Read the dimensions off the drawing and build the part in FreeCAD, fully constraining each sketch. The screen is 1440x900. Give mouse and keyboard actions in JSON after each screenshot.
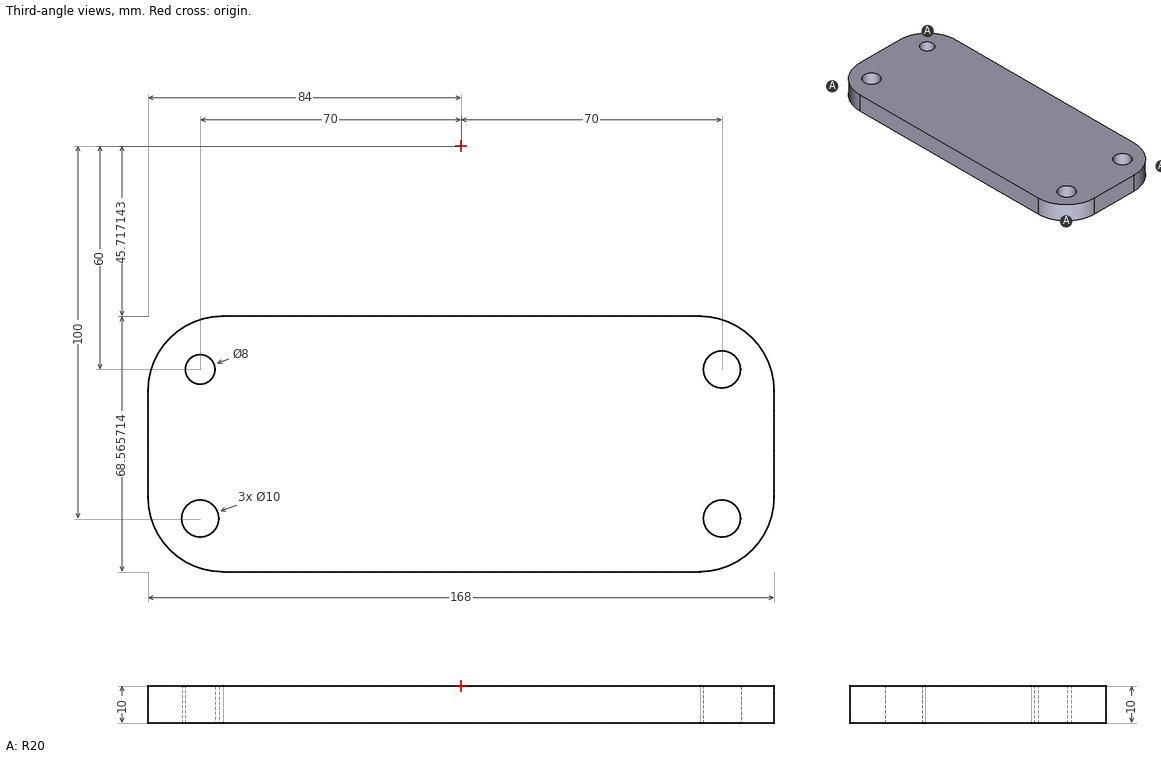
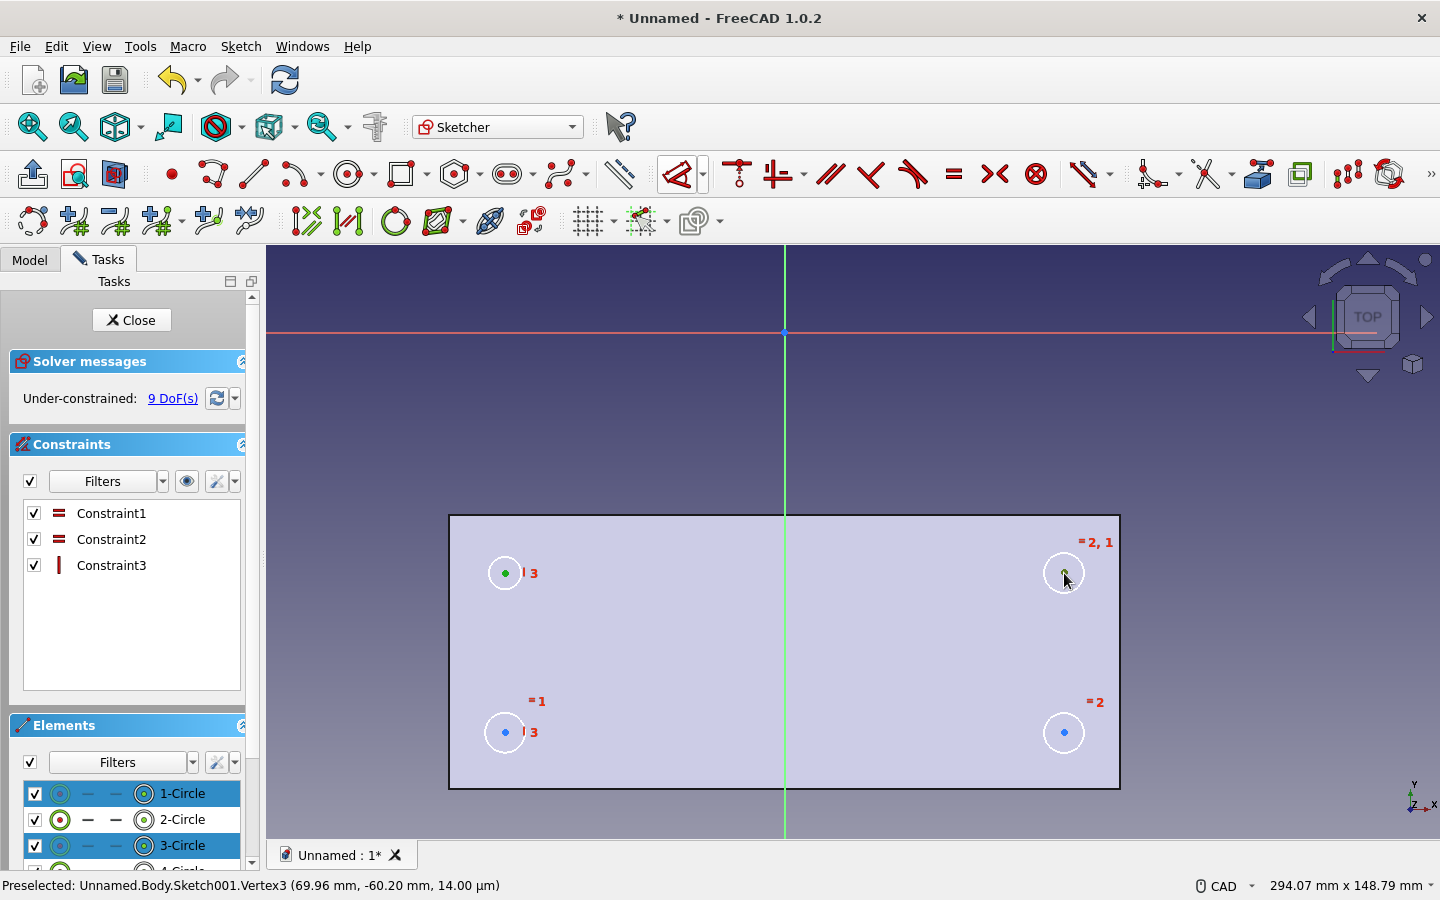
{"action": "key", "text": "h"}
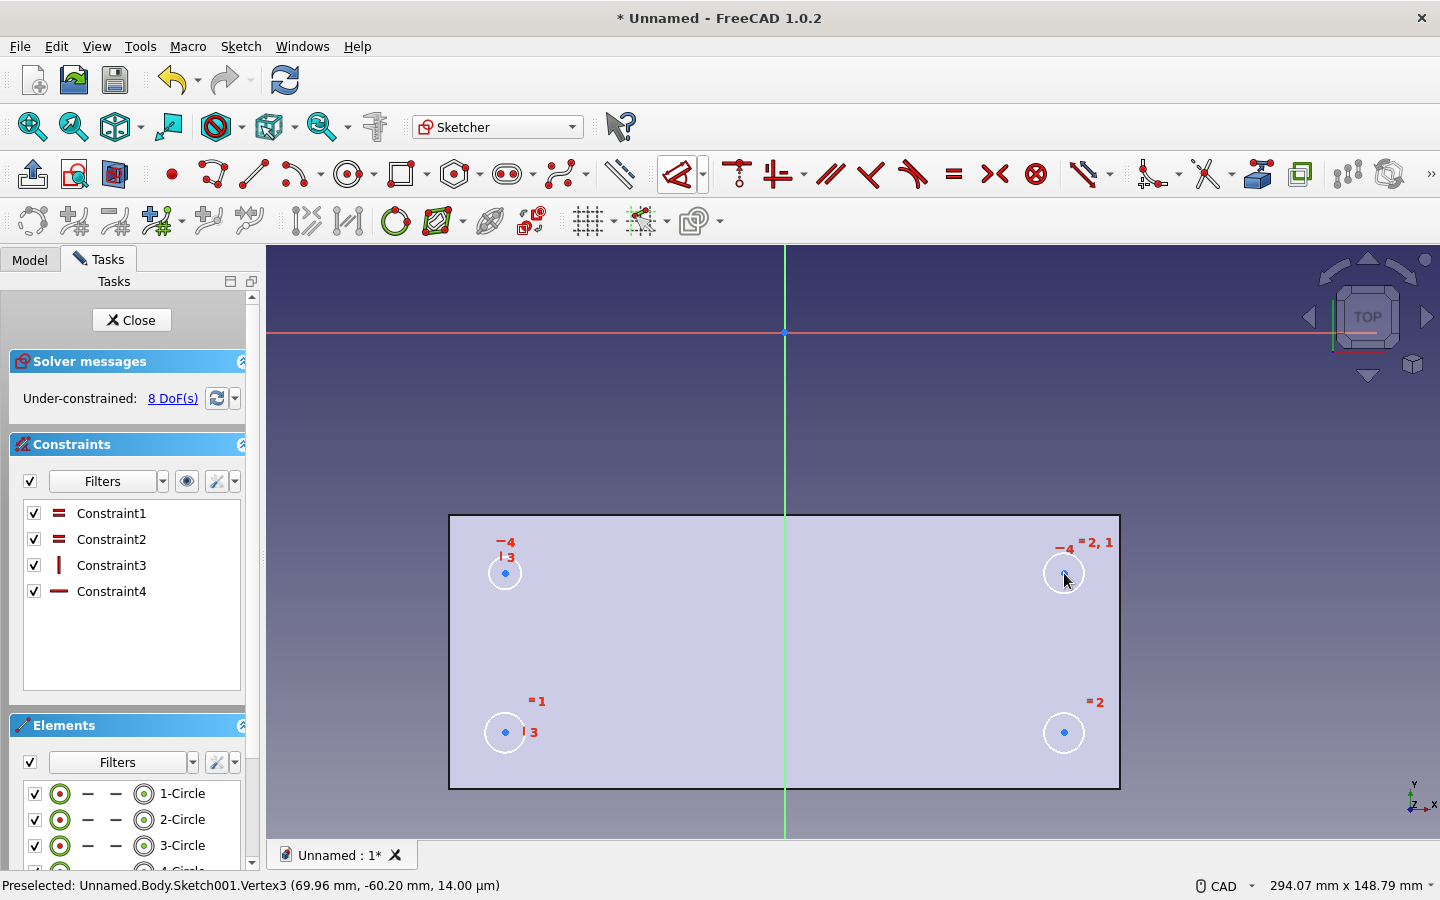
{"action": "left_click", "coordinate": [1064, 573]}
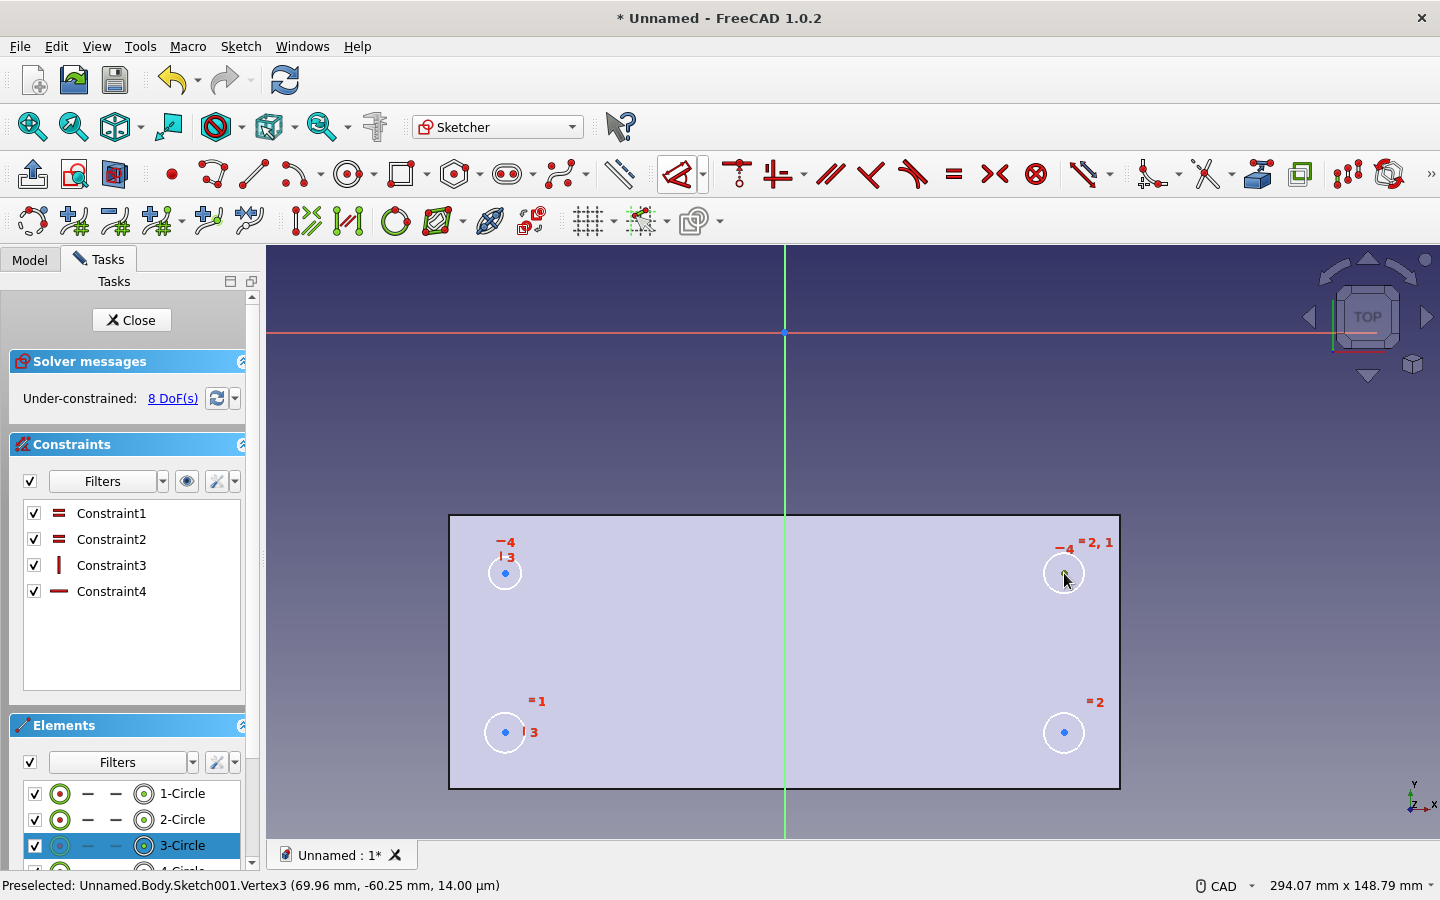
{"action": "left_click", "coordinate": [1064, 733]}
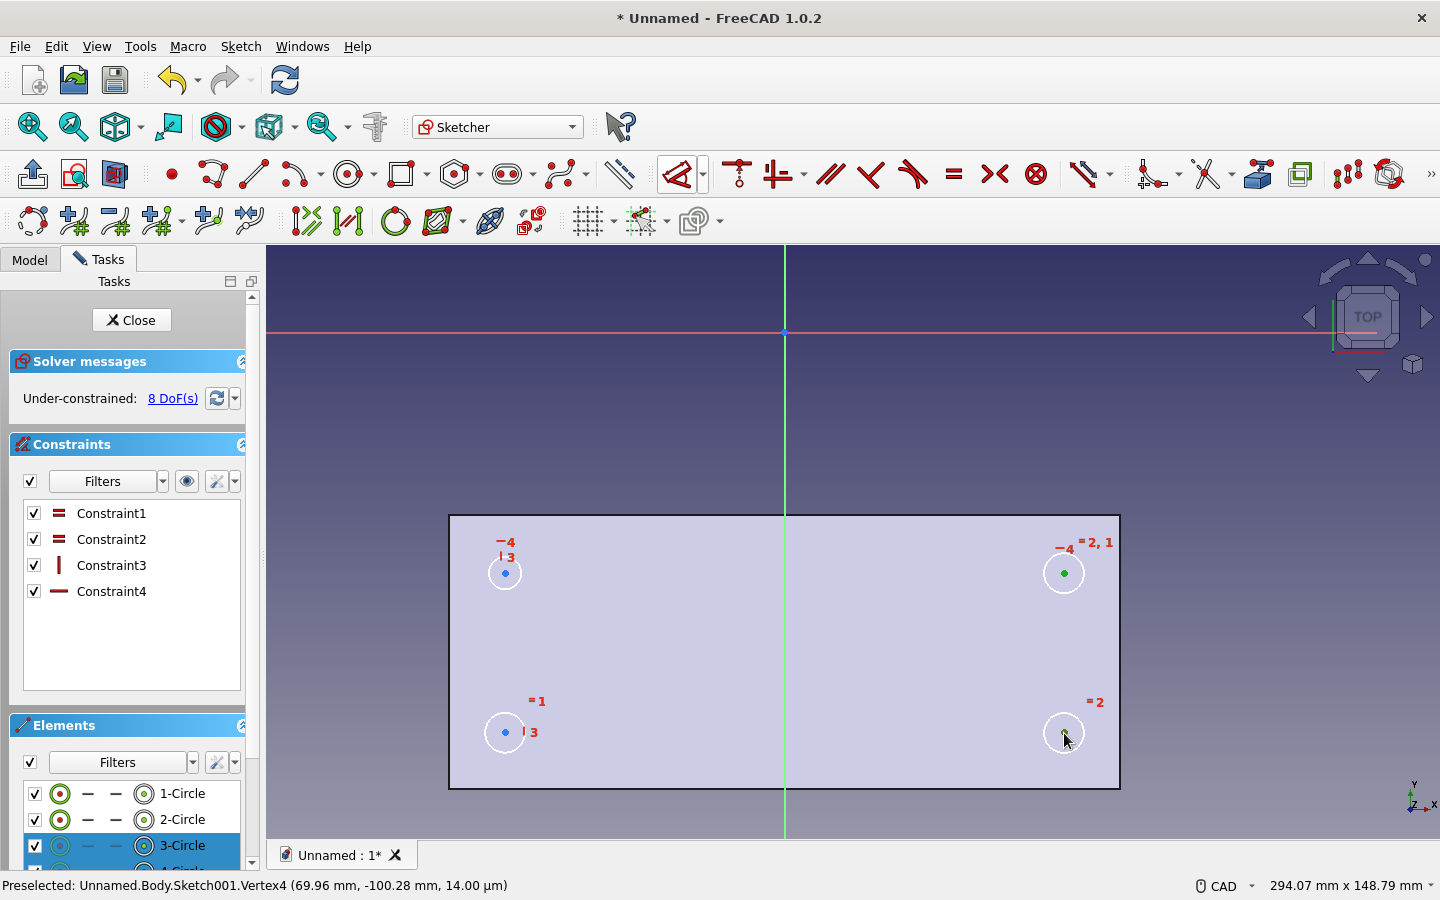
{"action": "key", "text": "v"}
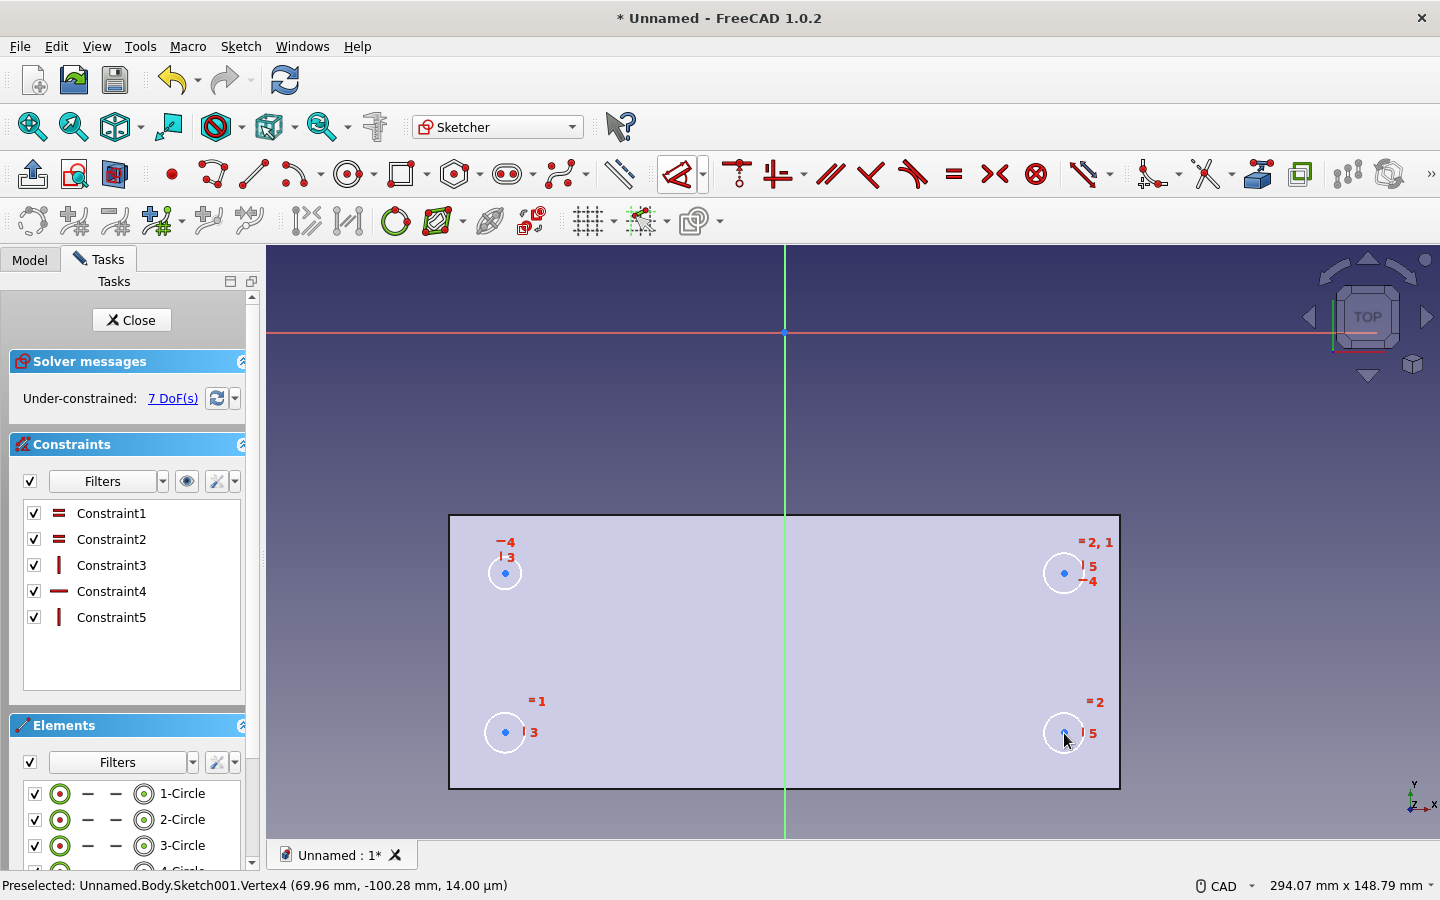
{"action": "left_click", "coordinate": [505, 733]}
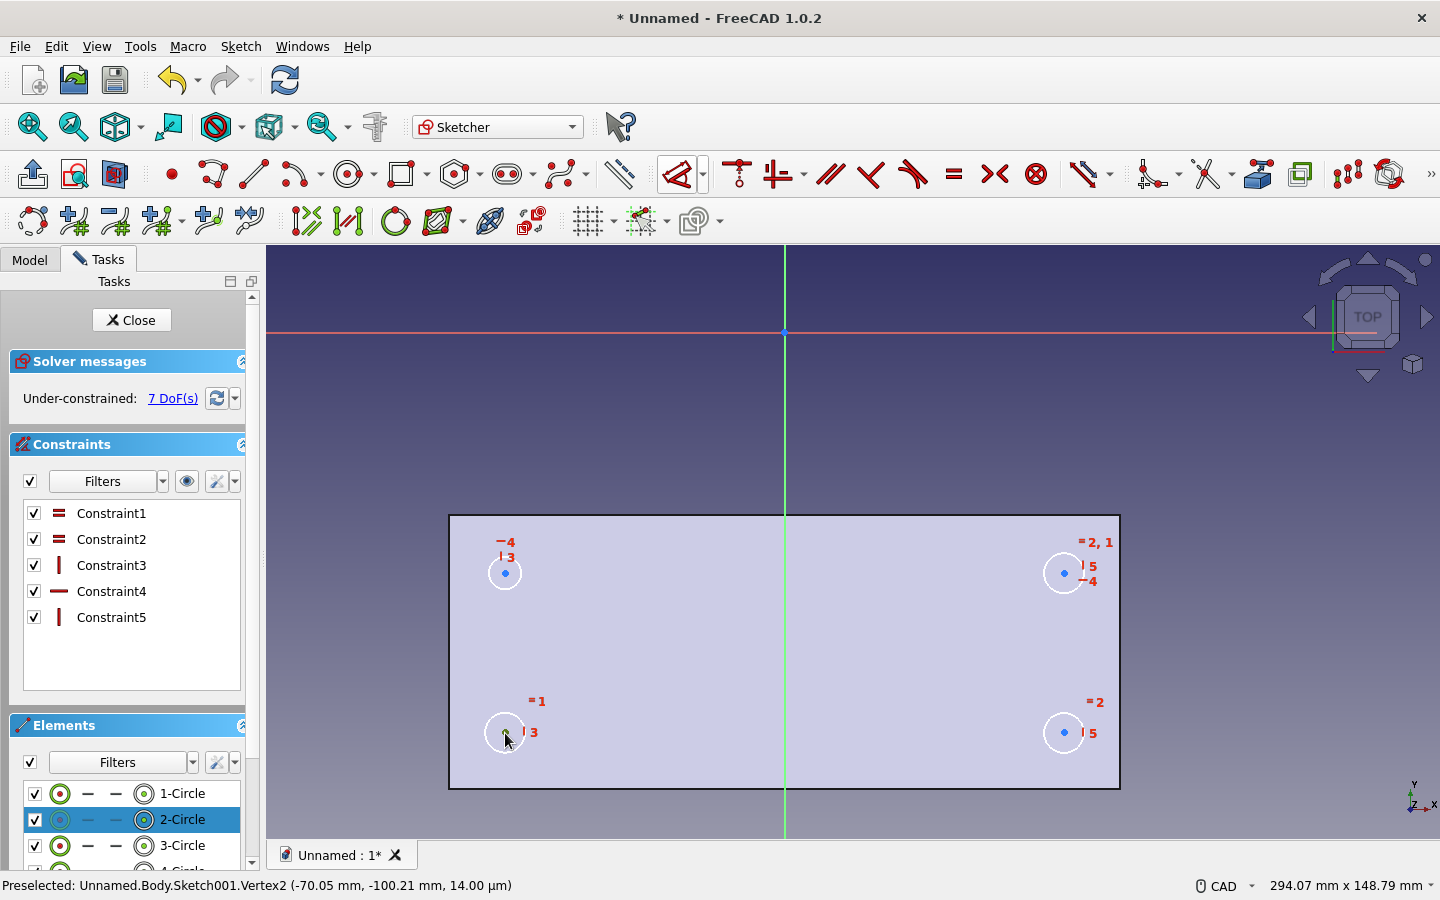
{"action": "left_click", "coordinate": [1064, 733]}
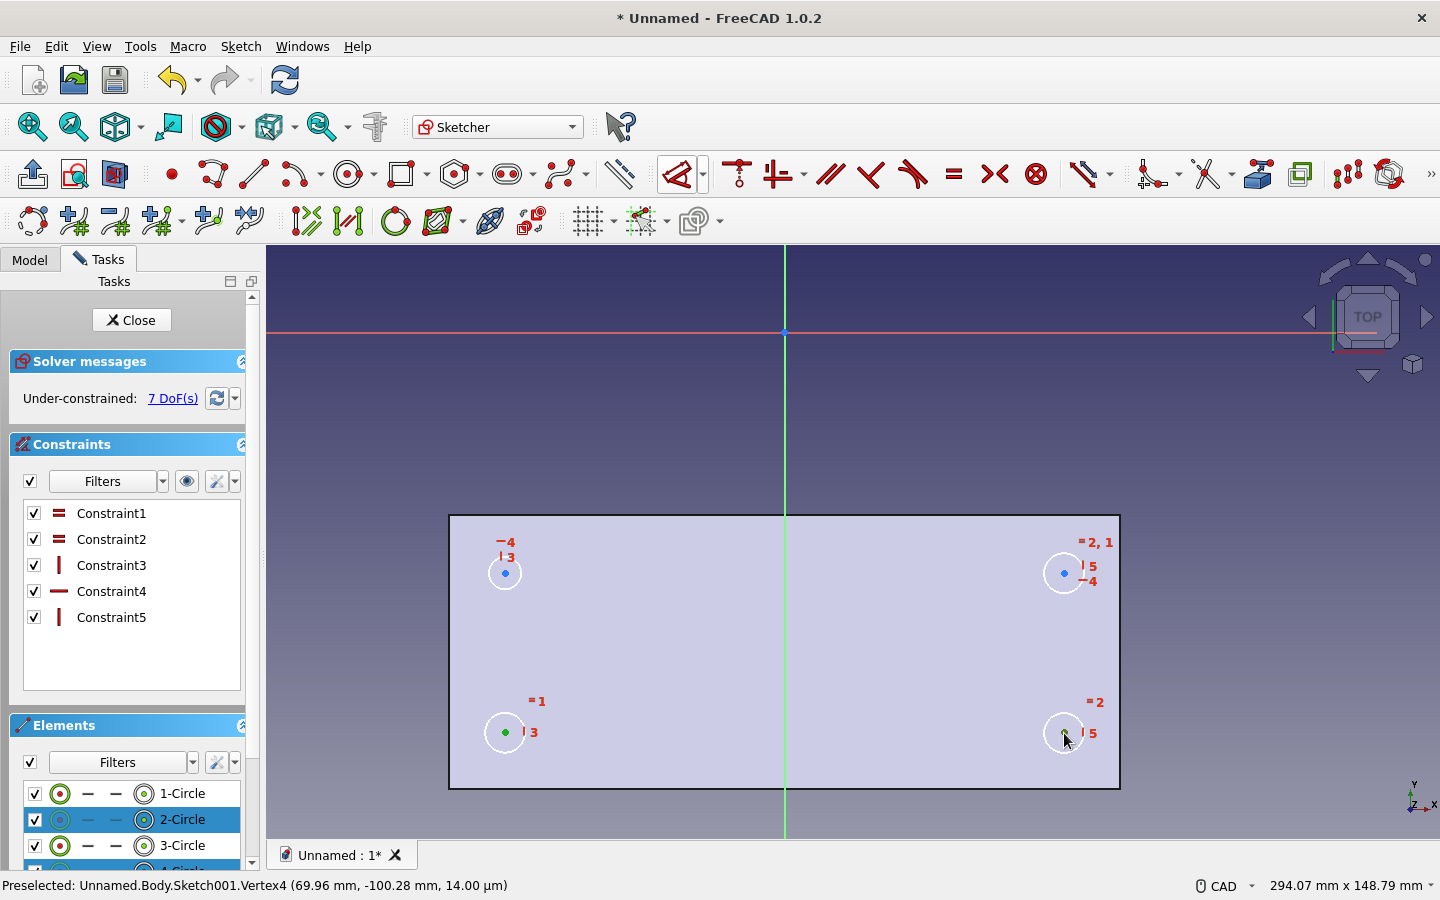
{"action": "left_click", "coordinate": [804, 174]}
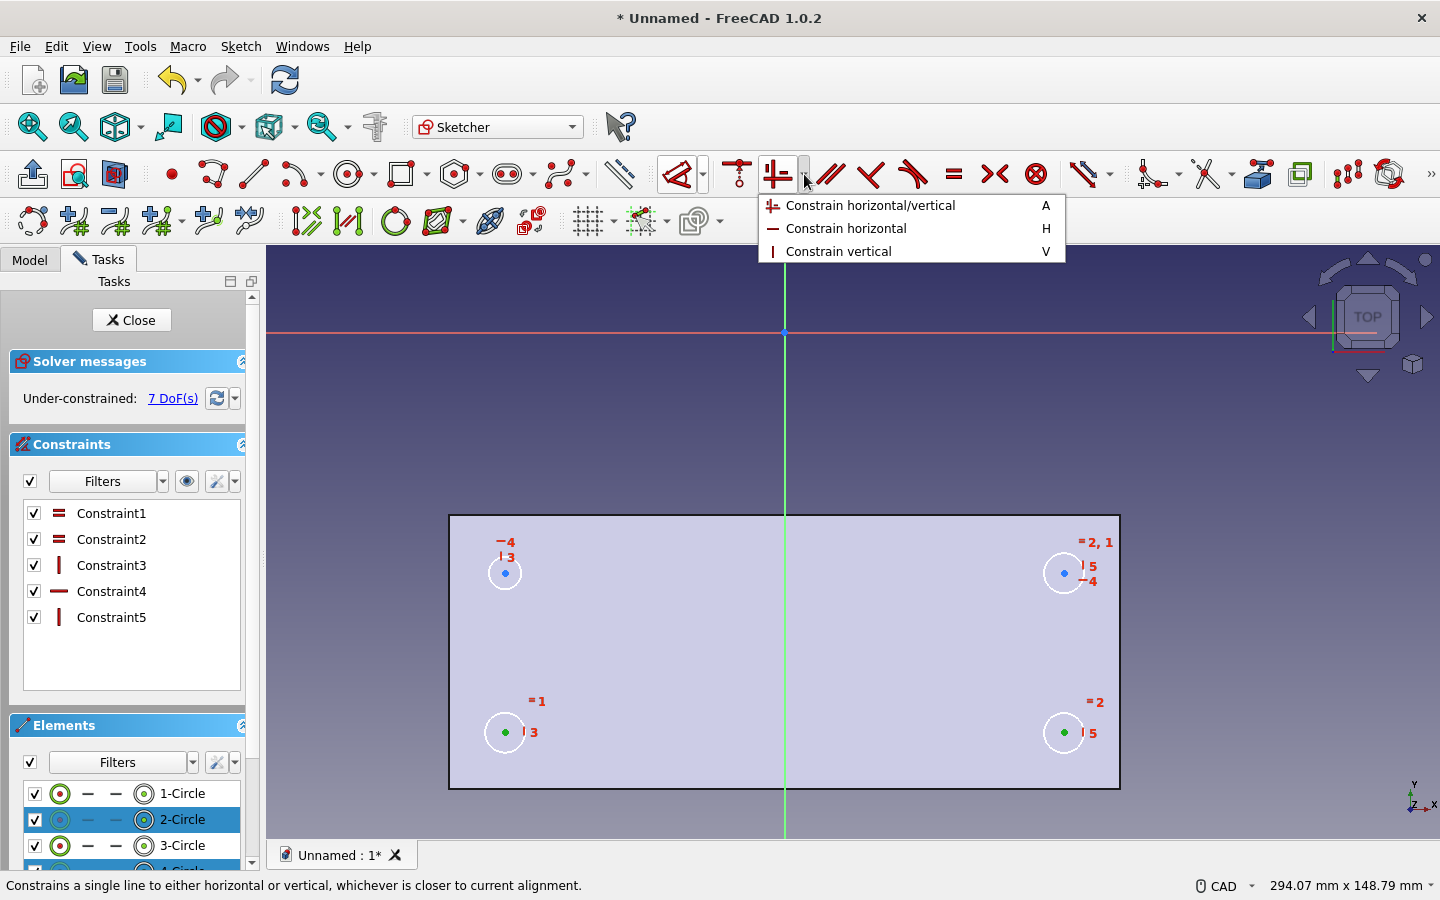
{"action": "left_click", "coordinate": [912, 228]}